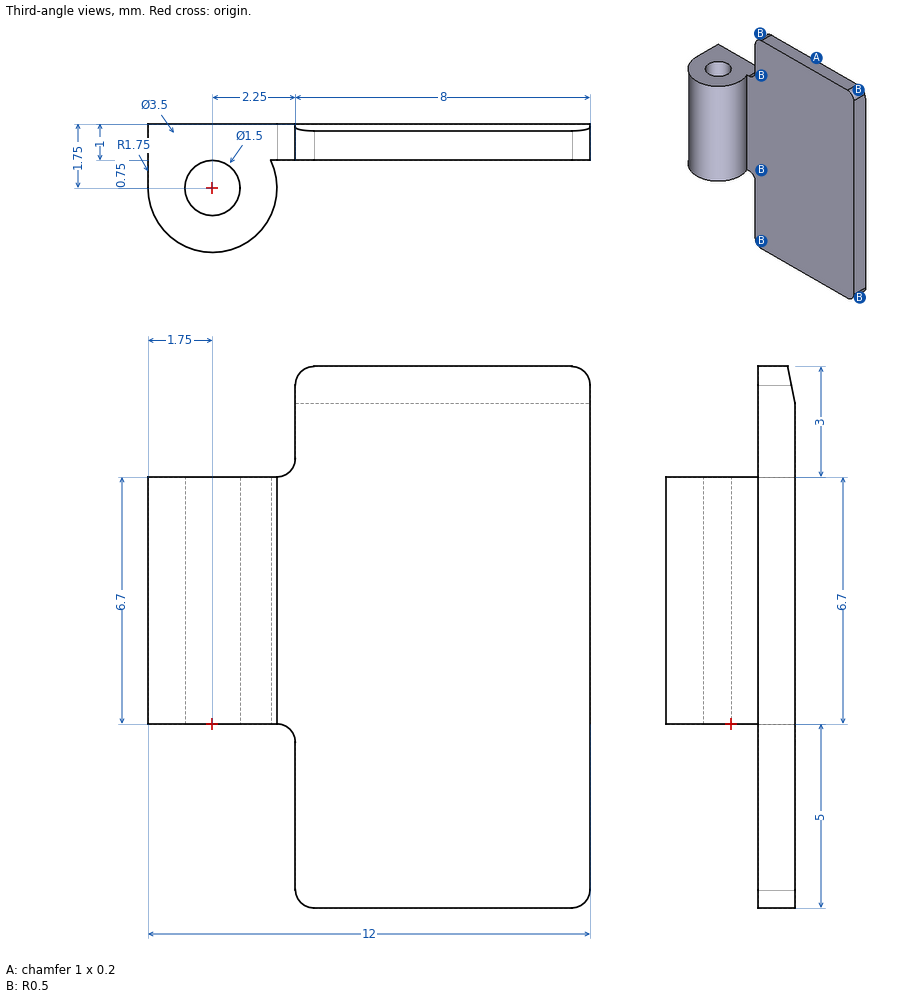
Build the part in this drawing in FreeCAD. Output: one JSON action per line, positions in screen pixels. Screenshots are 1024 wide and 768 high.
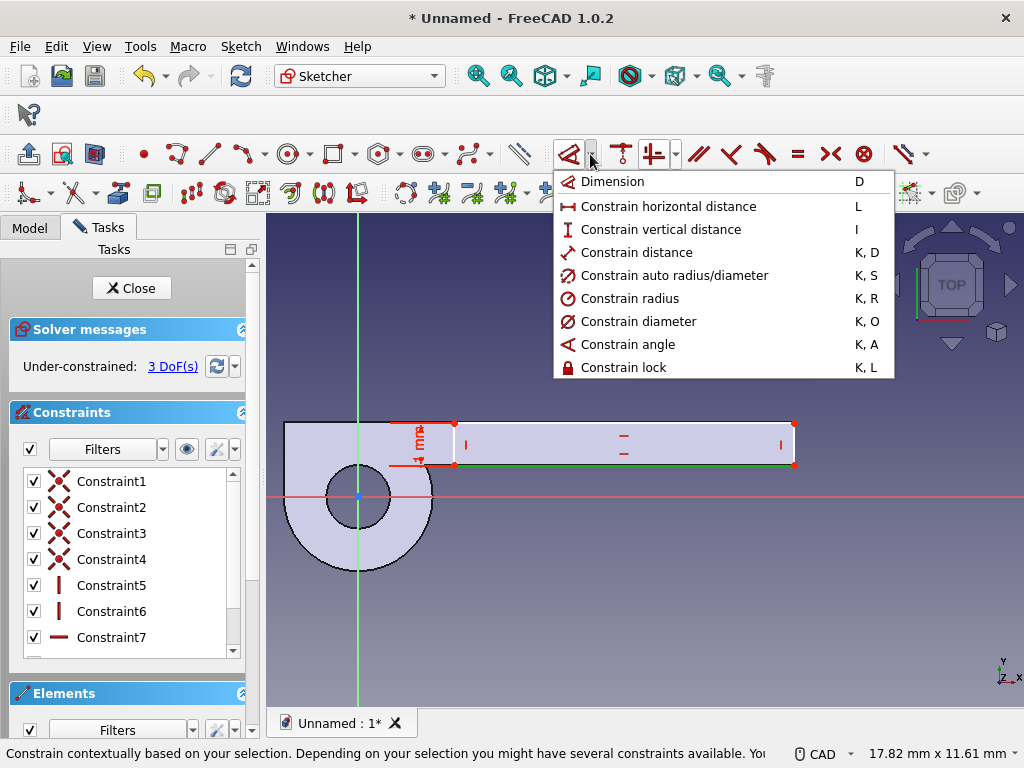
{"action": "left_click", "coordinate": [724, 206]}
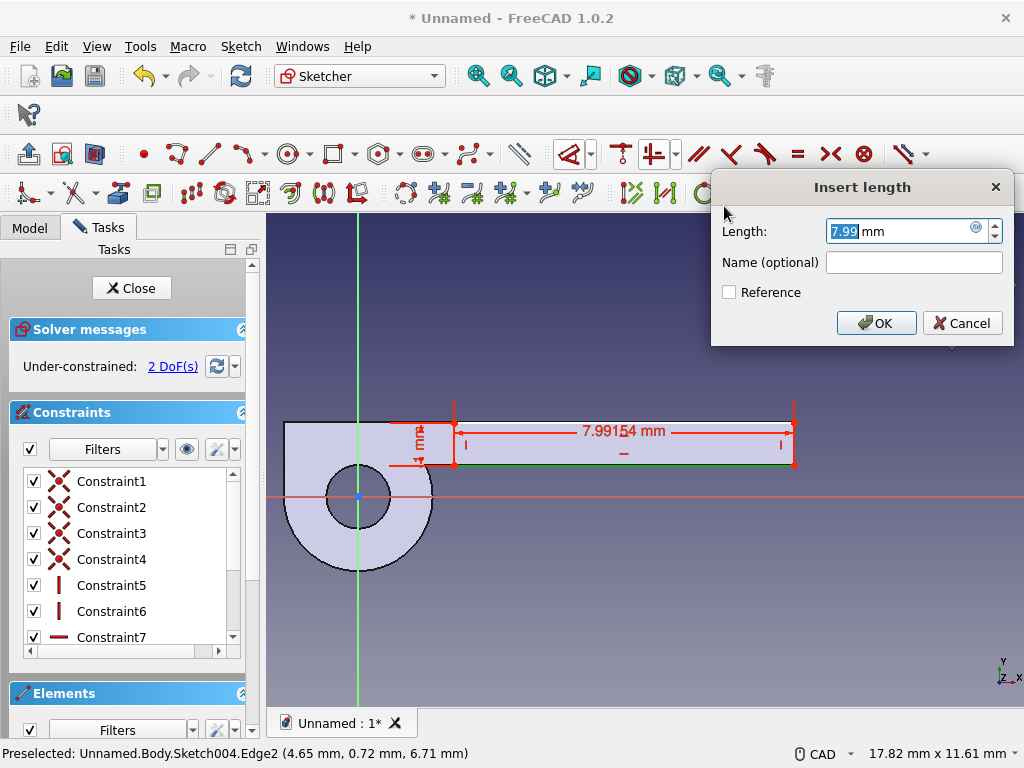
{"action": "type", "text": "8"}
{"action": "key", "text": "Return"}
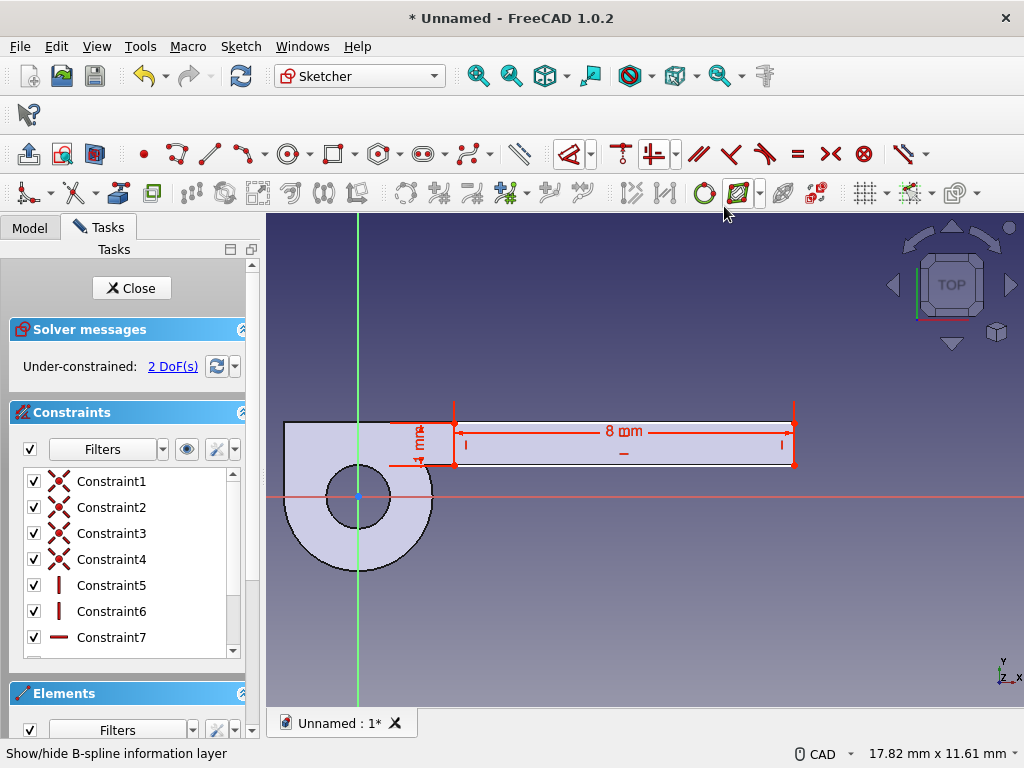
{"action": "left_click", "coordinate": [454, 423]}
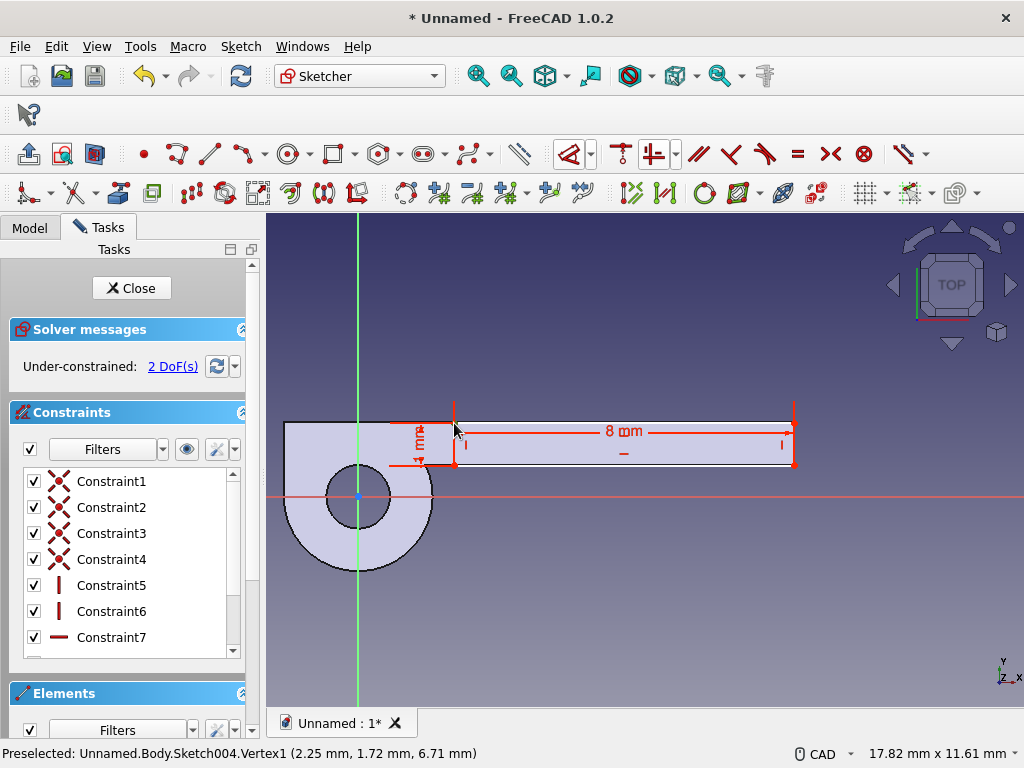
{"action": "left_click", "coordinate": [590, 154]}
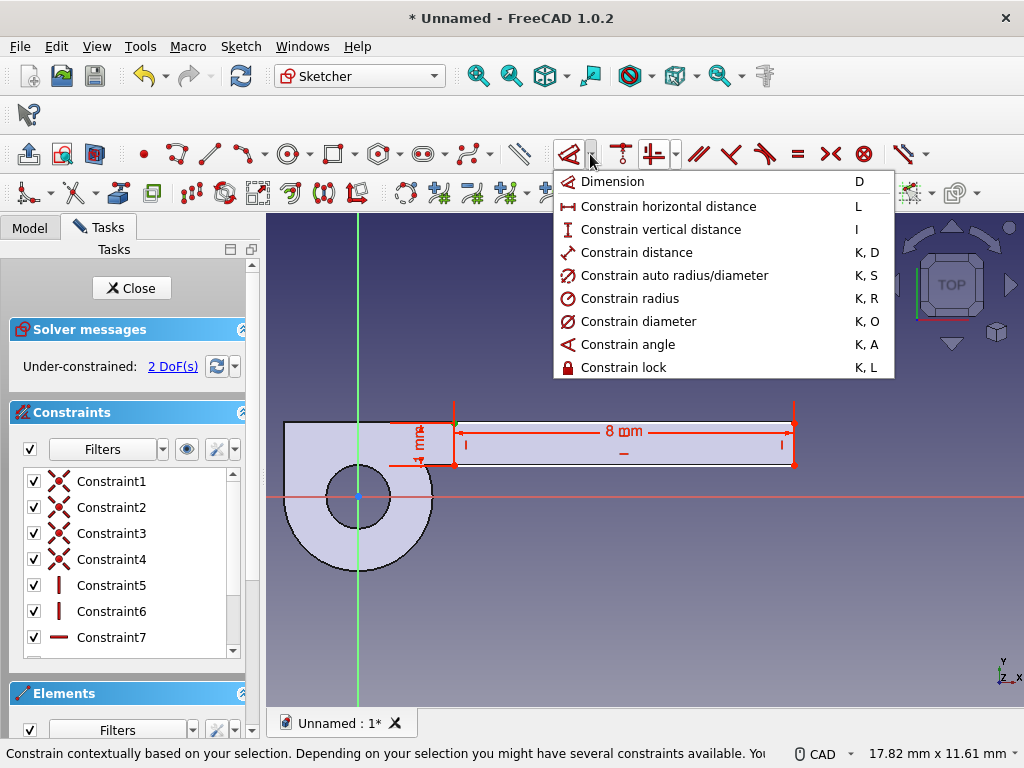
{"action": "left_click", "coordinate": [724, 206]}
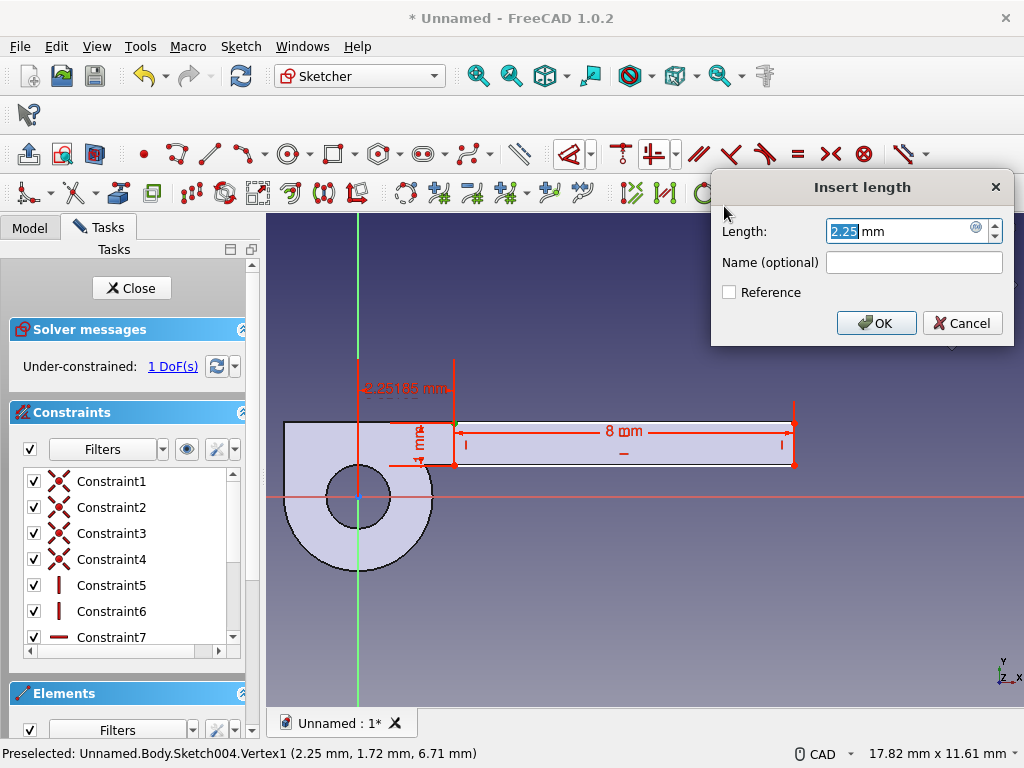
{"action": "type", "text": "2.25"}
{"action": "key", "text": "Return"}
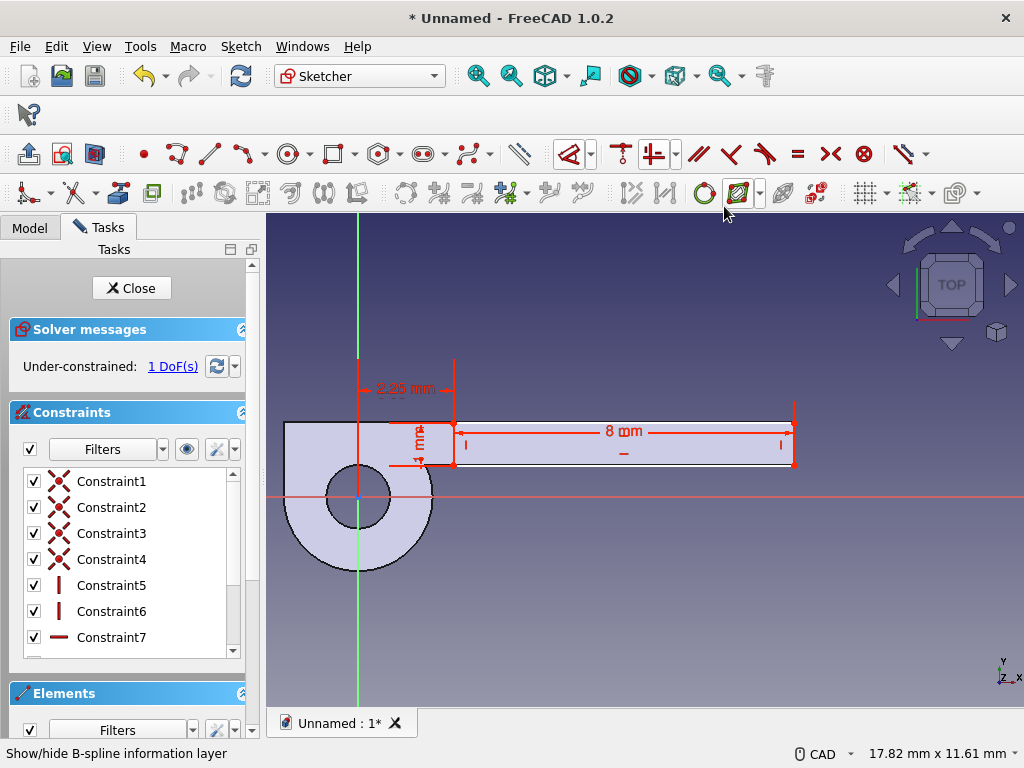
{"action": "left_click", "coordinate": [454, 423]}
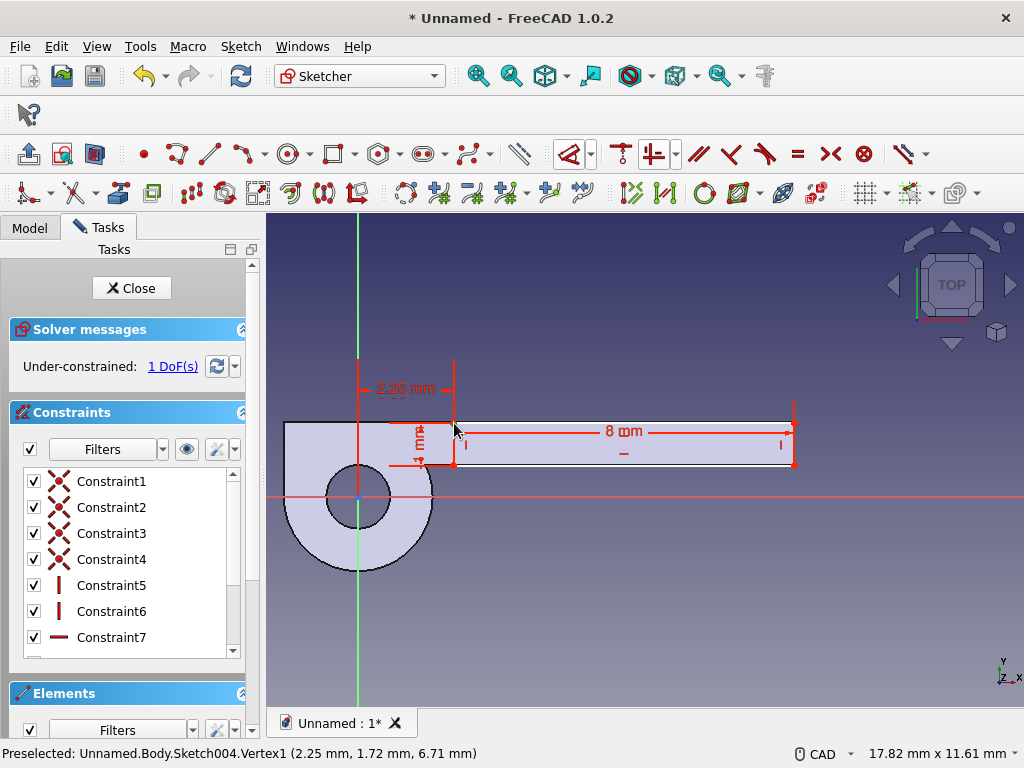
{"action": "left_click", "coordinate": [590, 154]}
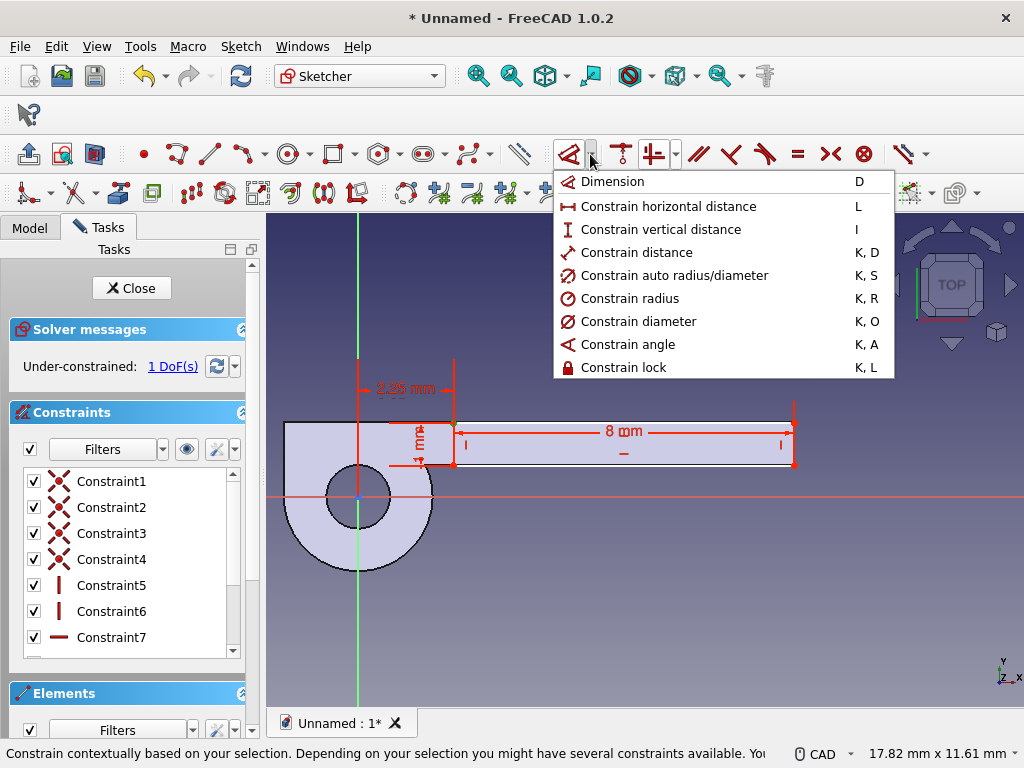
{"action": "left_click", "coordinate": [724, 230]}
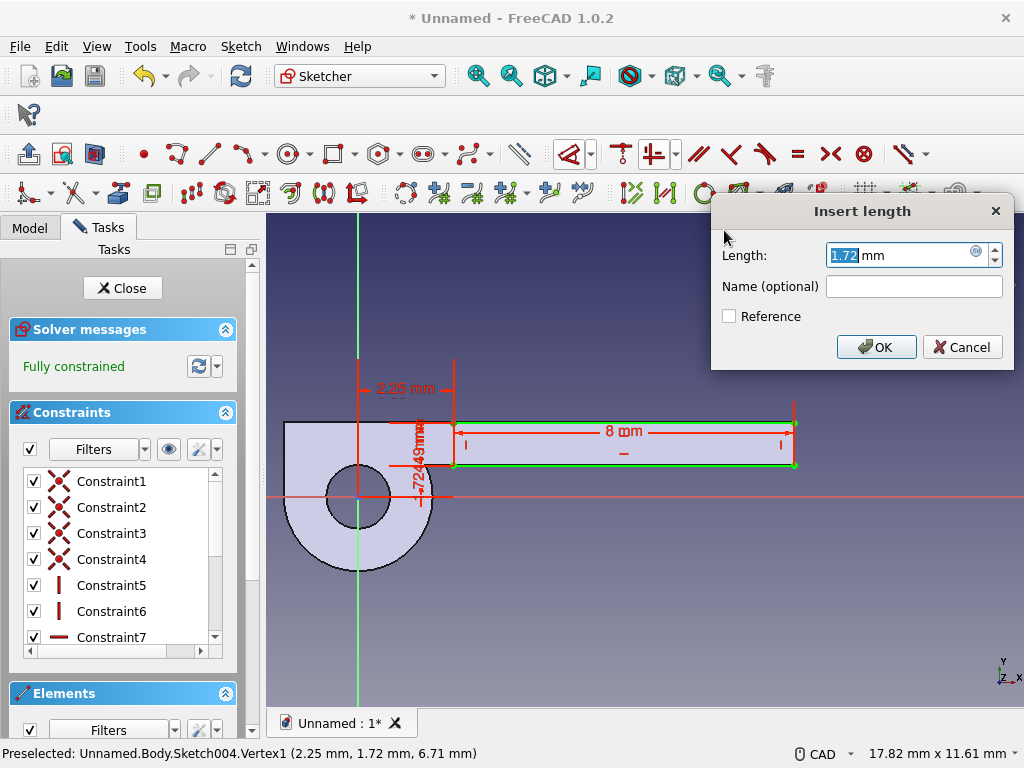
{"action": "type", "text": "1.75"}
{"action": "key", "text": "Return"}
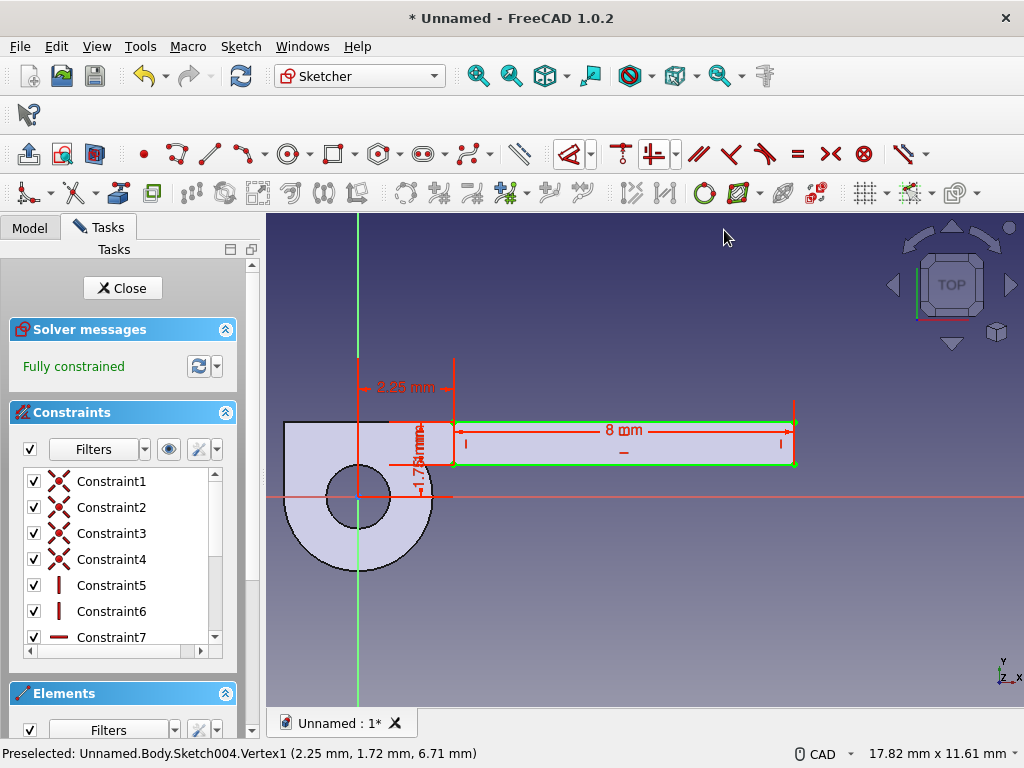
{"action": "left_click", "coordinate": [123, 288]}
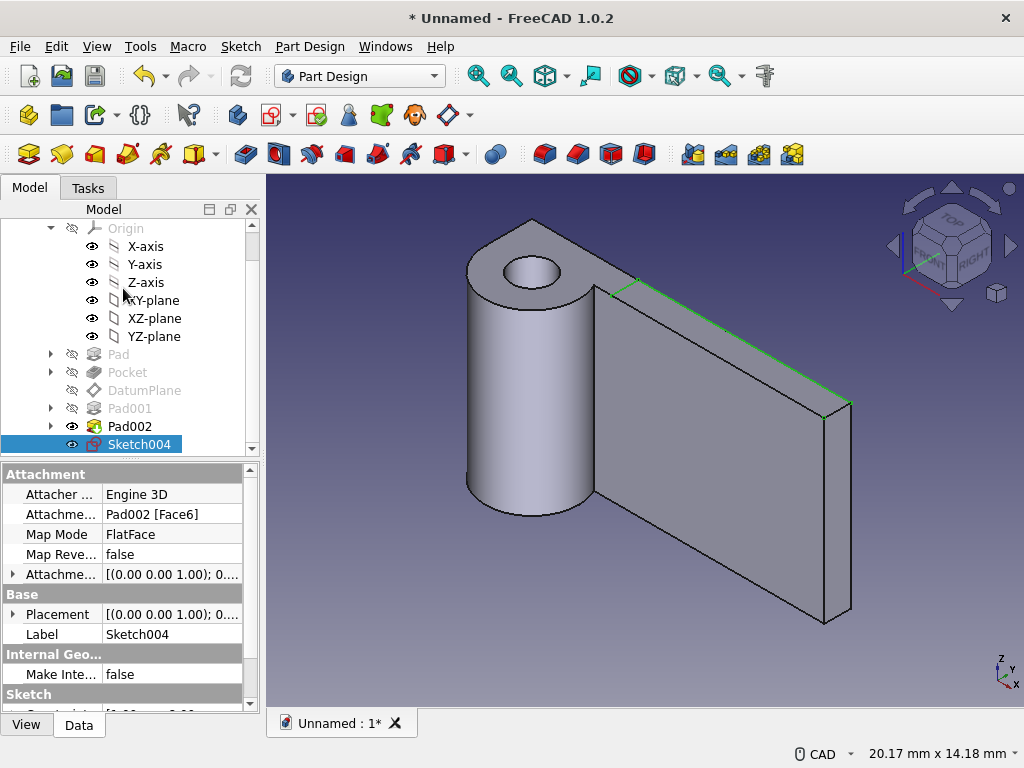
{"action": "left_click", "coordinate": [29, 154]}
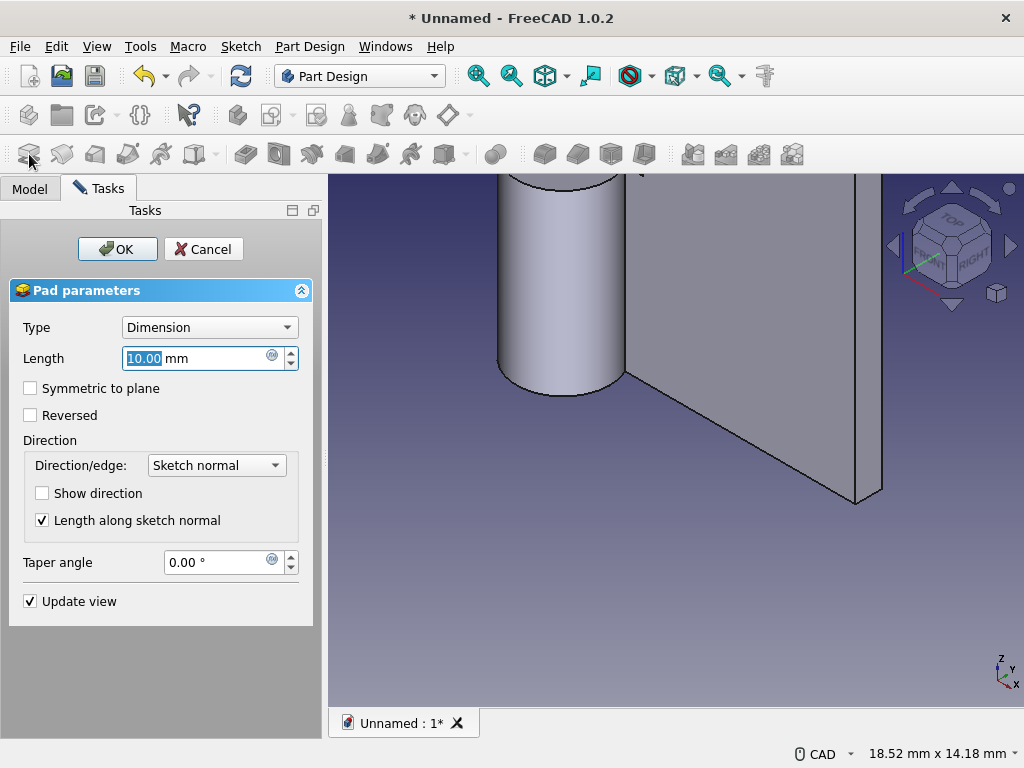
{"action": "type", "text": "3"}
{"action": "key", "text": "Tab"}